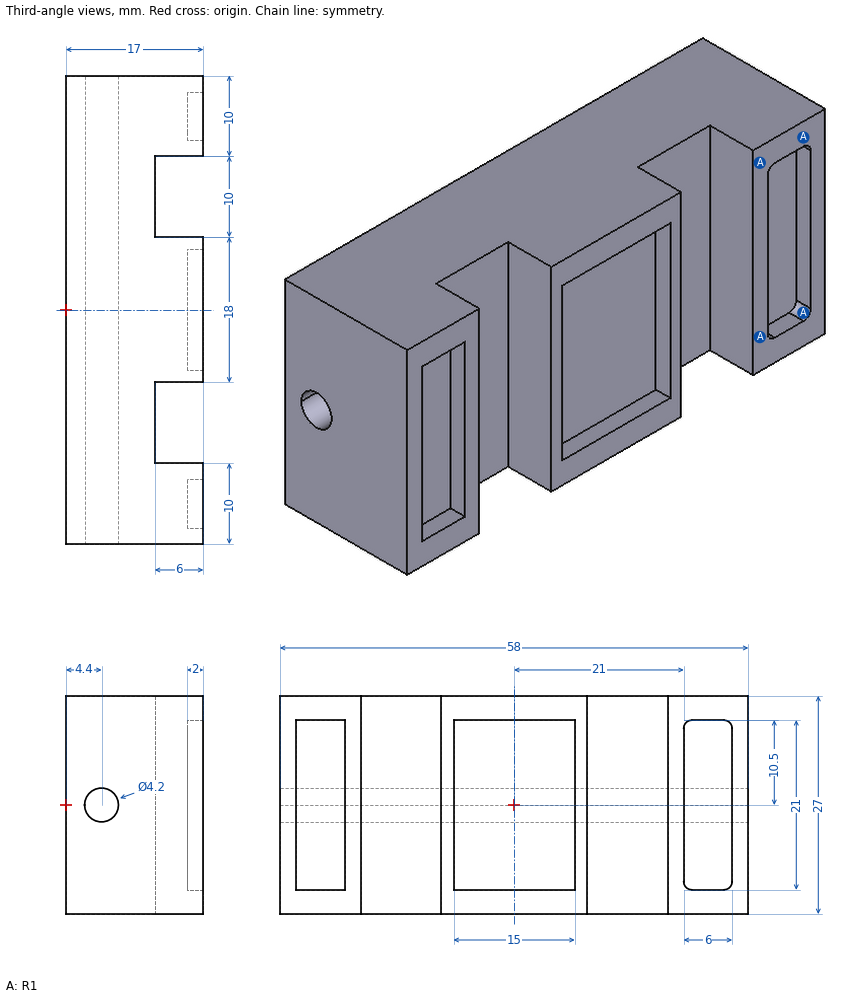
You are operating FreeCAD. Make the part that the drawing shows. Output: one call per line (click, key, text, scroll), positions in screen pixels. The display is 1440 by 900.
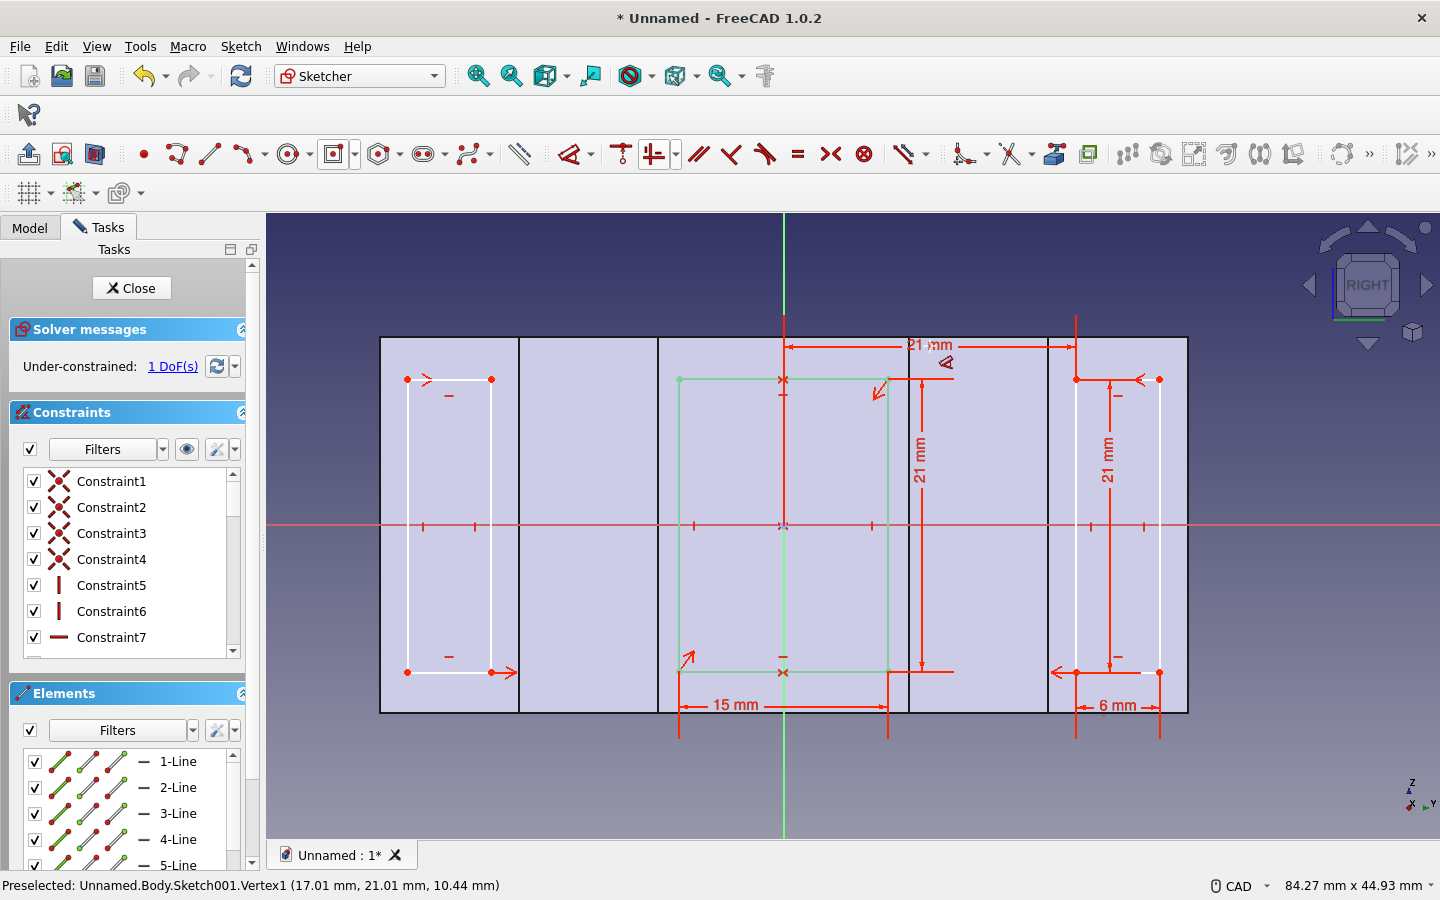
click(1076, 380)
click(1110, 419)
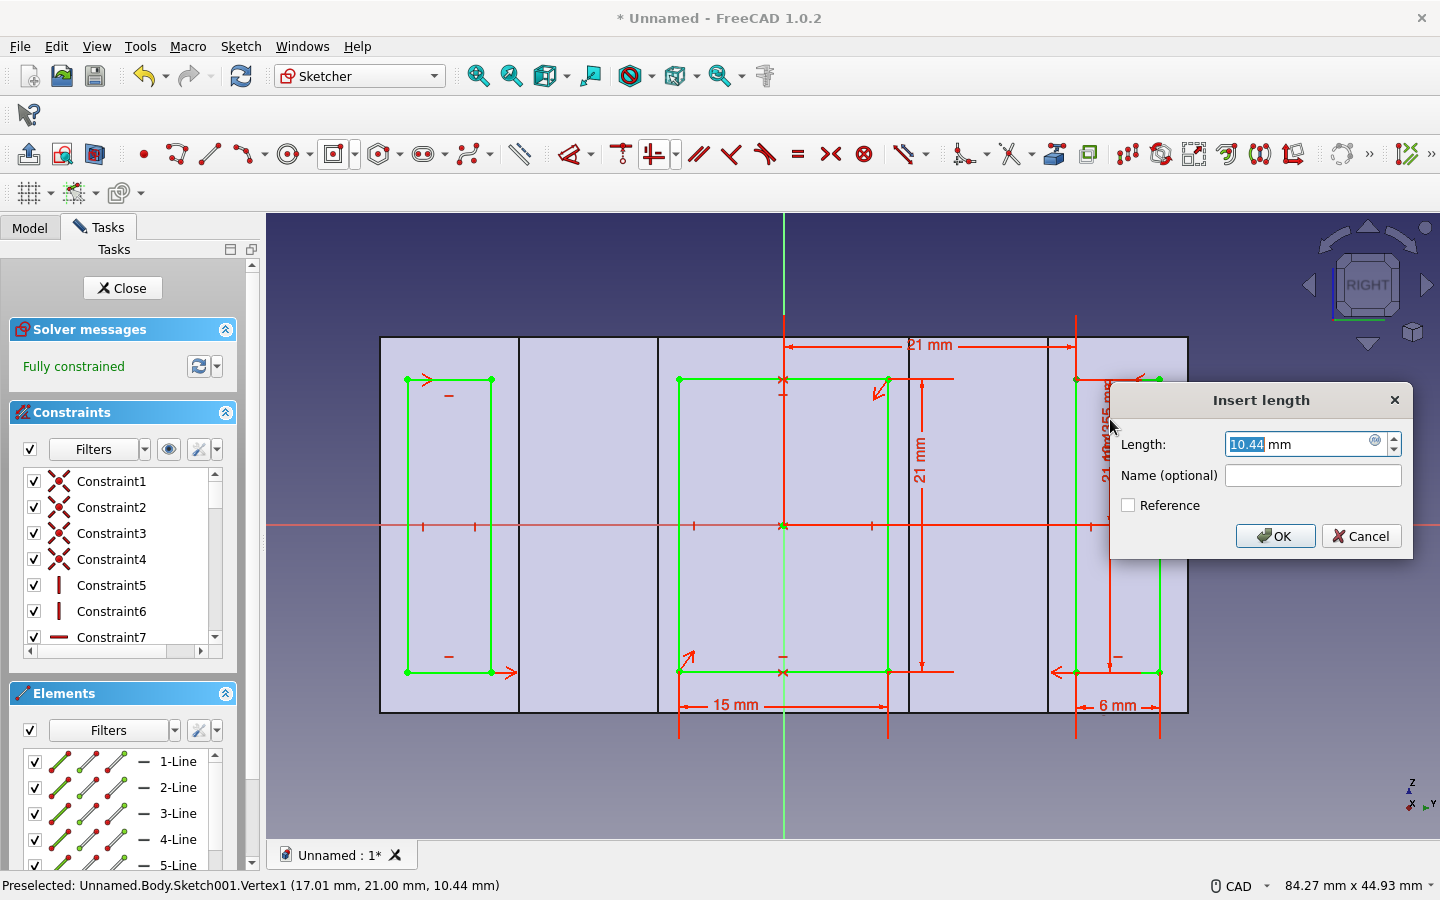
text(10.5)
key(Return)
key(Escape)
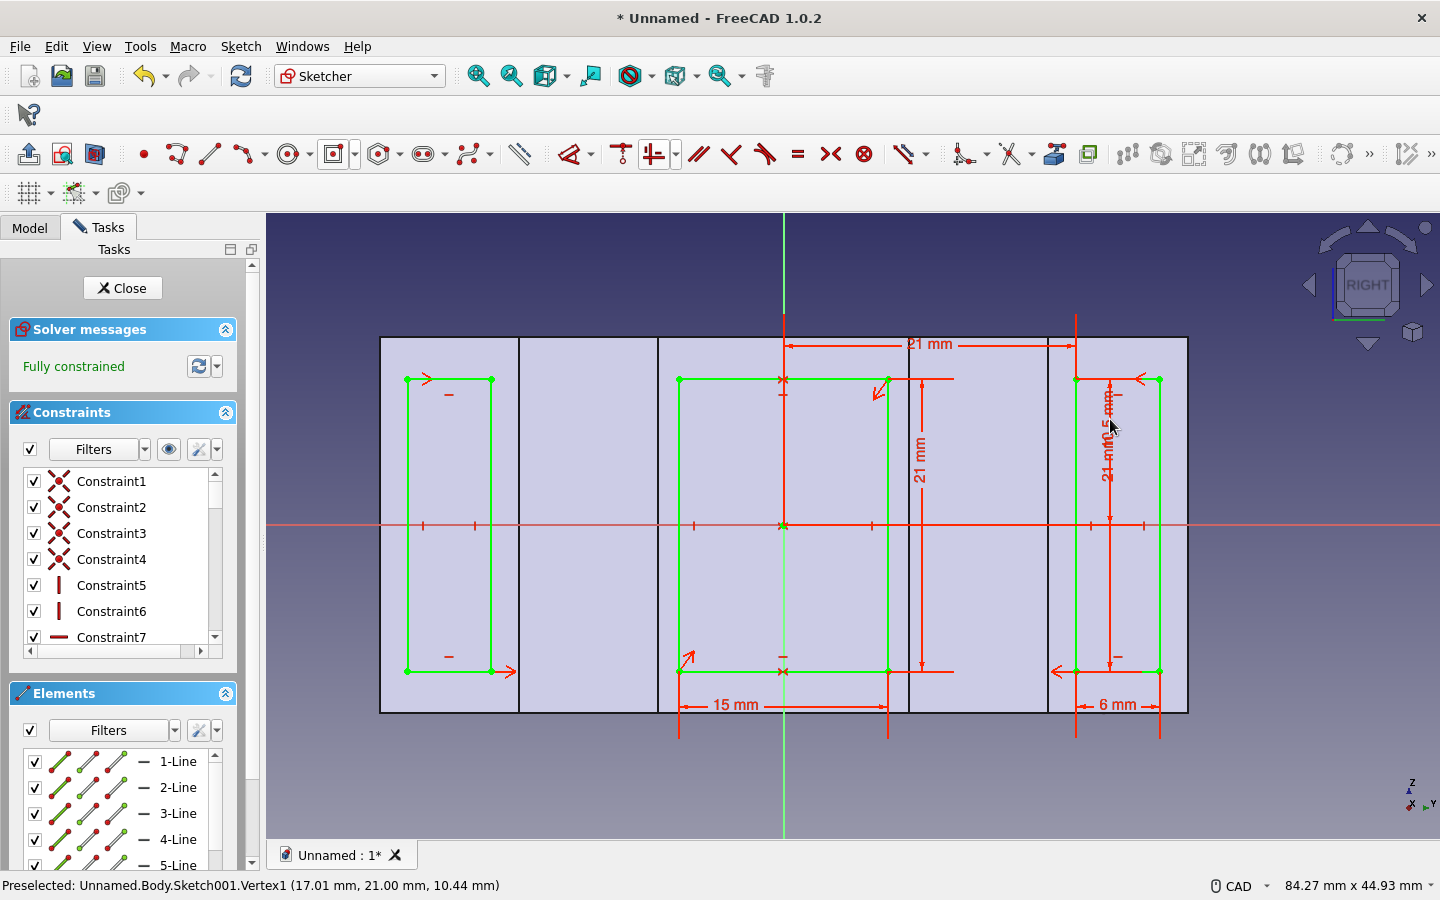
click(123, 288)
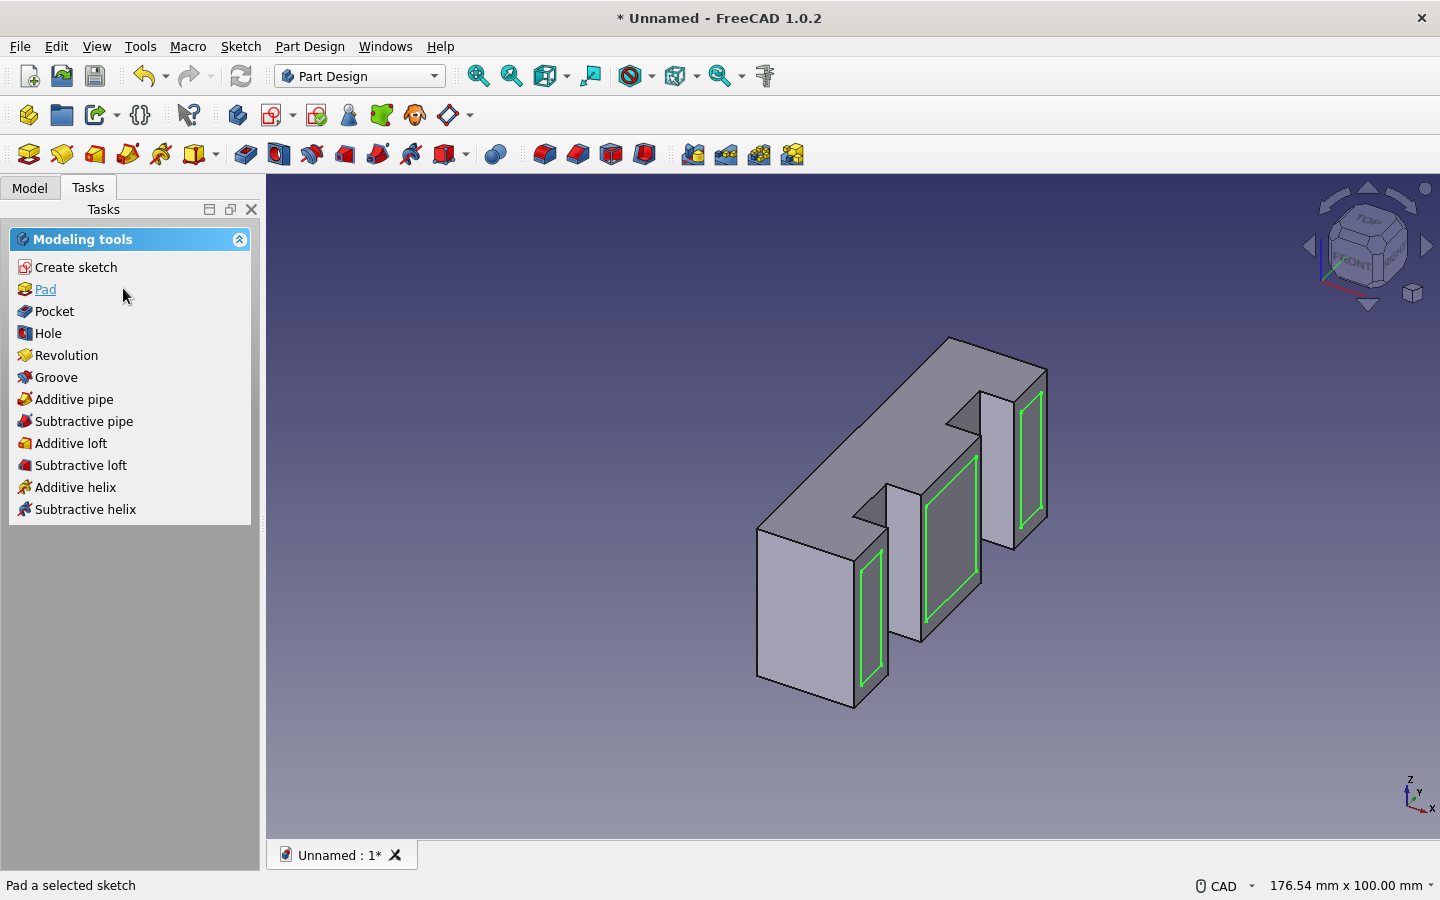
click(246, 154)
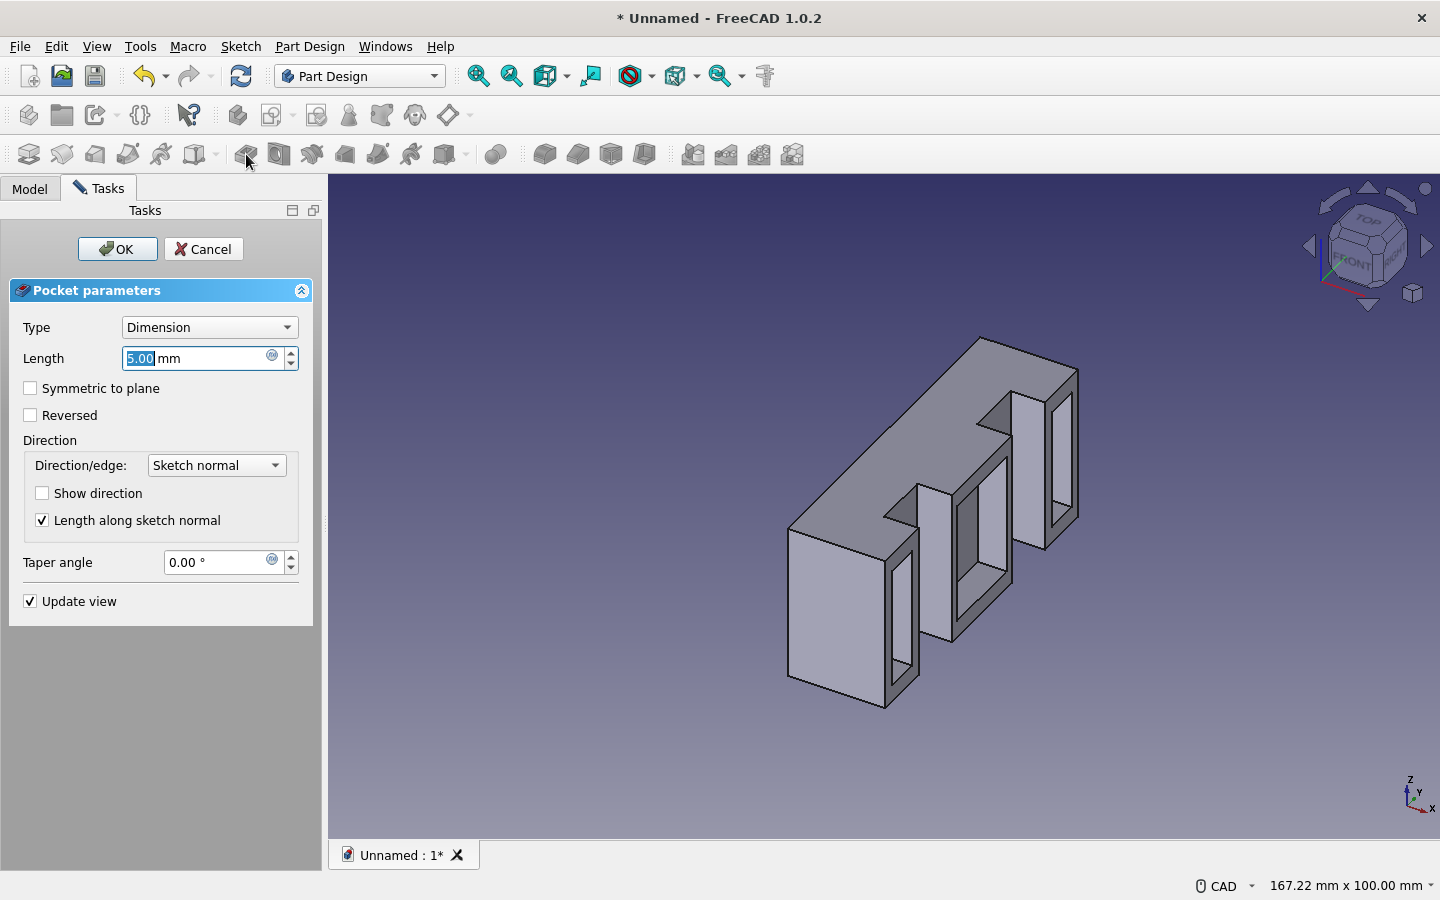
text(2)
key(Tab)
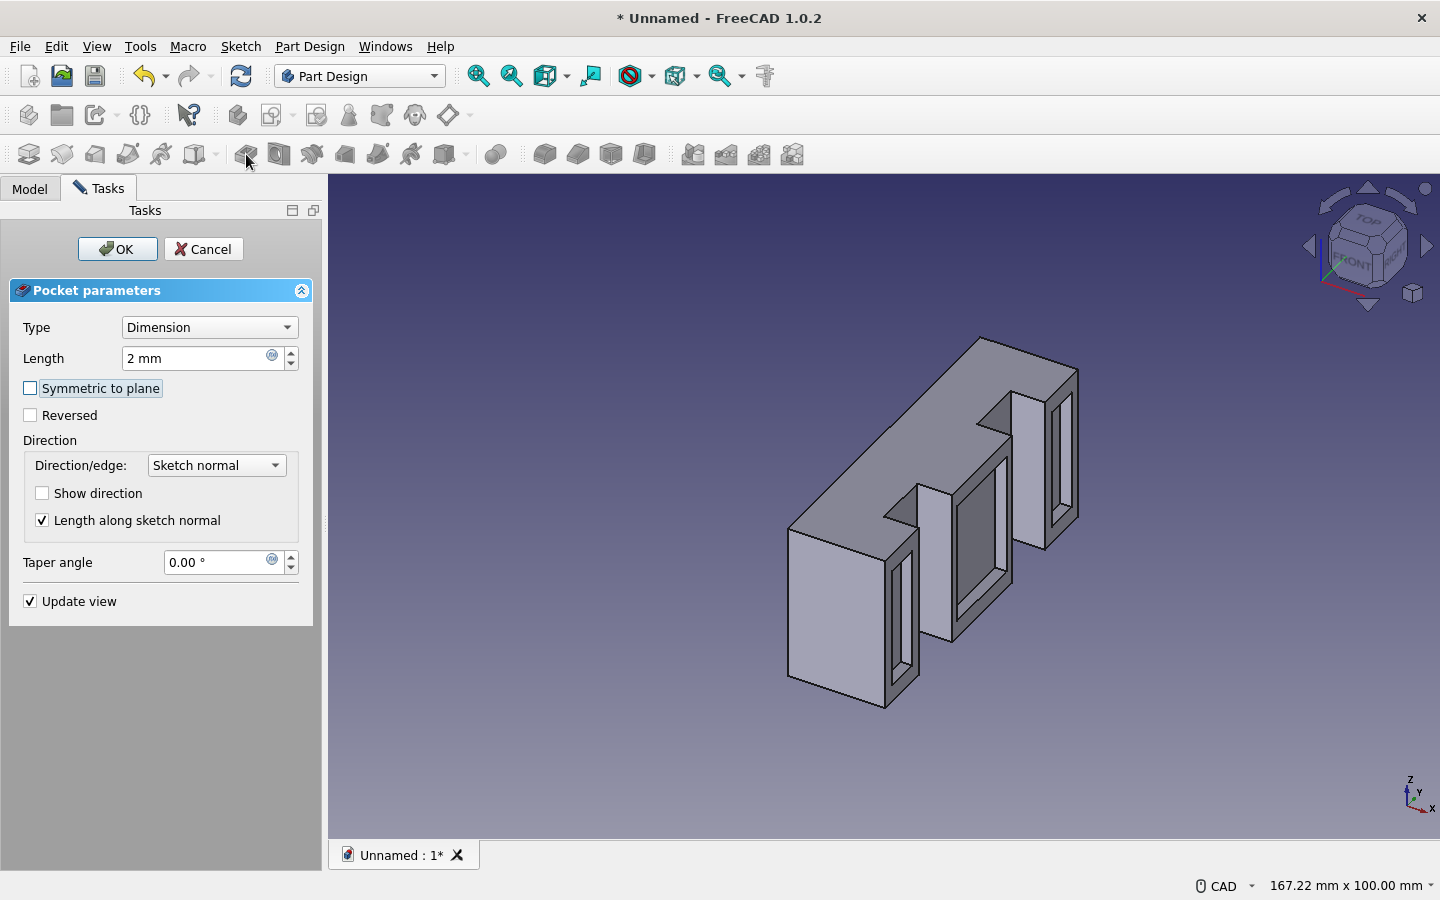
click(118, 249)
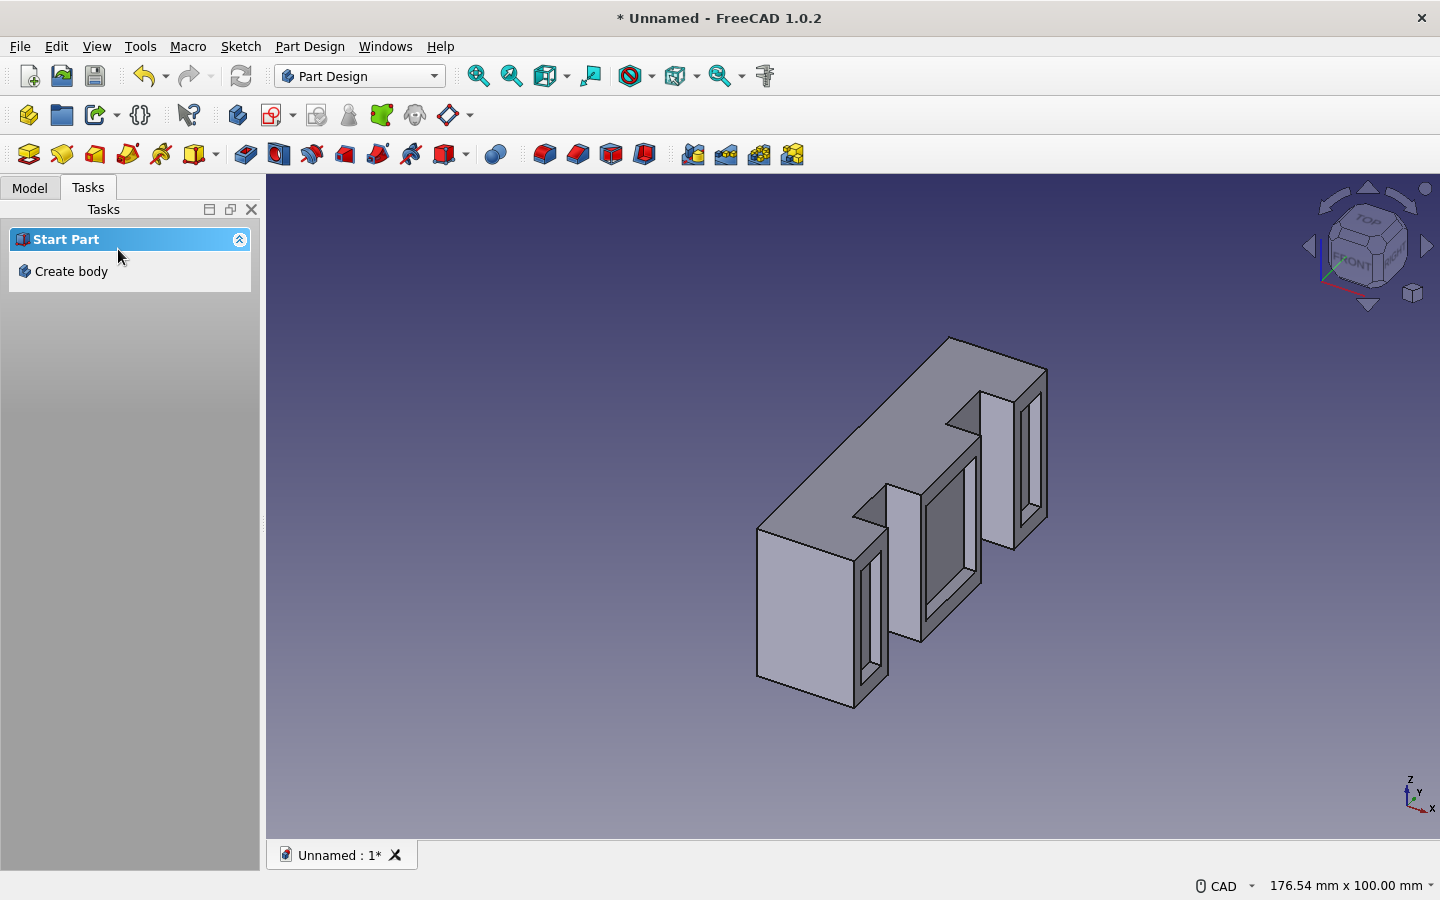
scroll(1035, 504, up, 6)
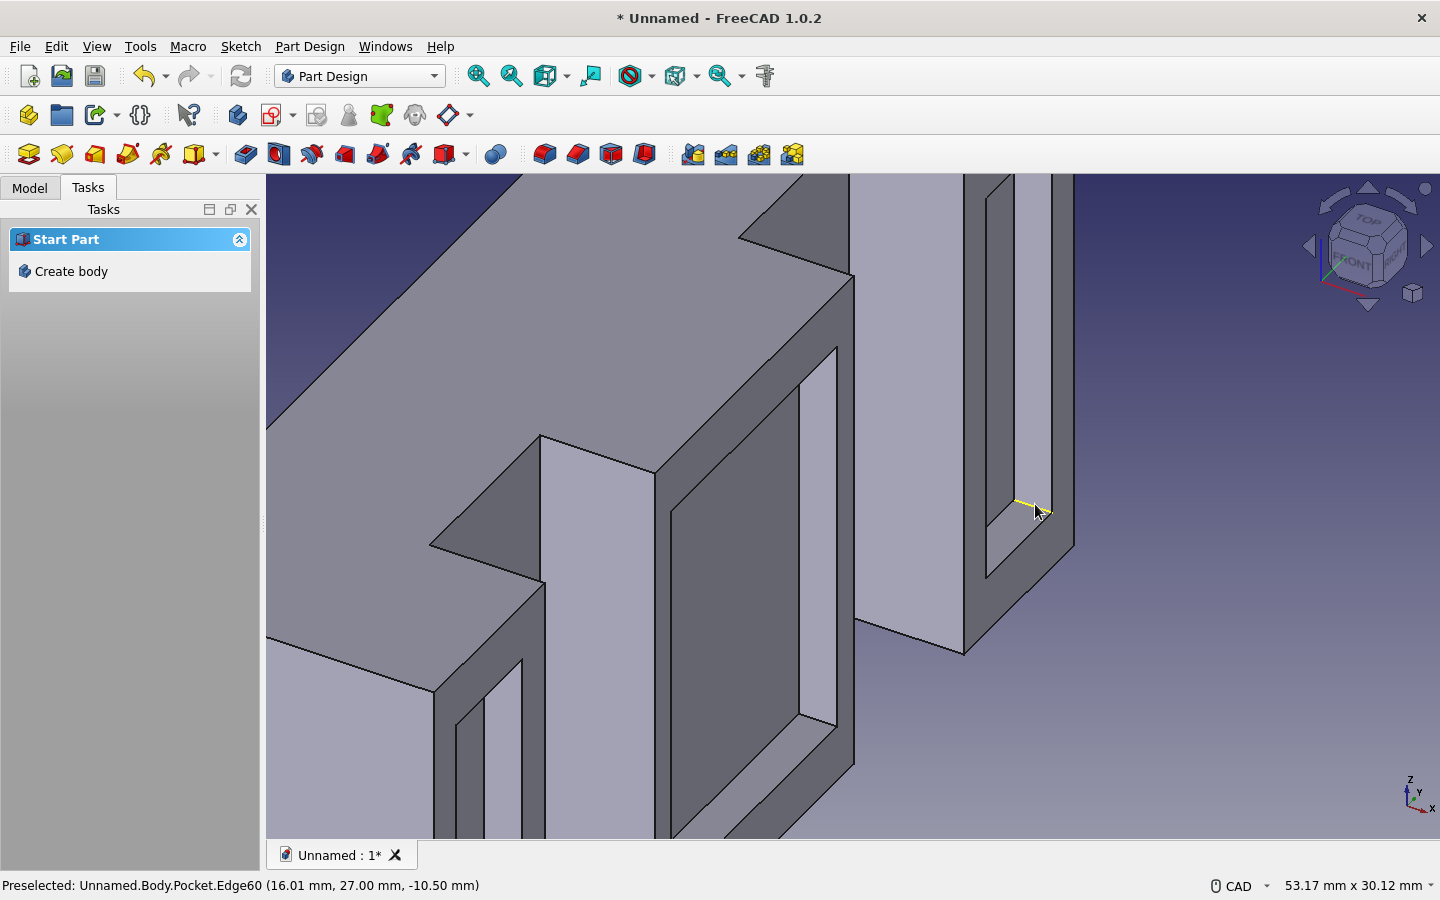
click(479, 76)